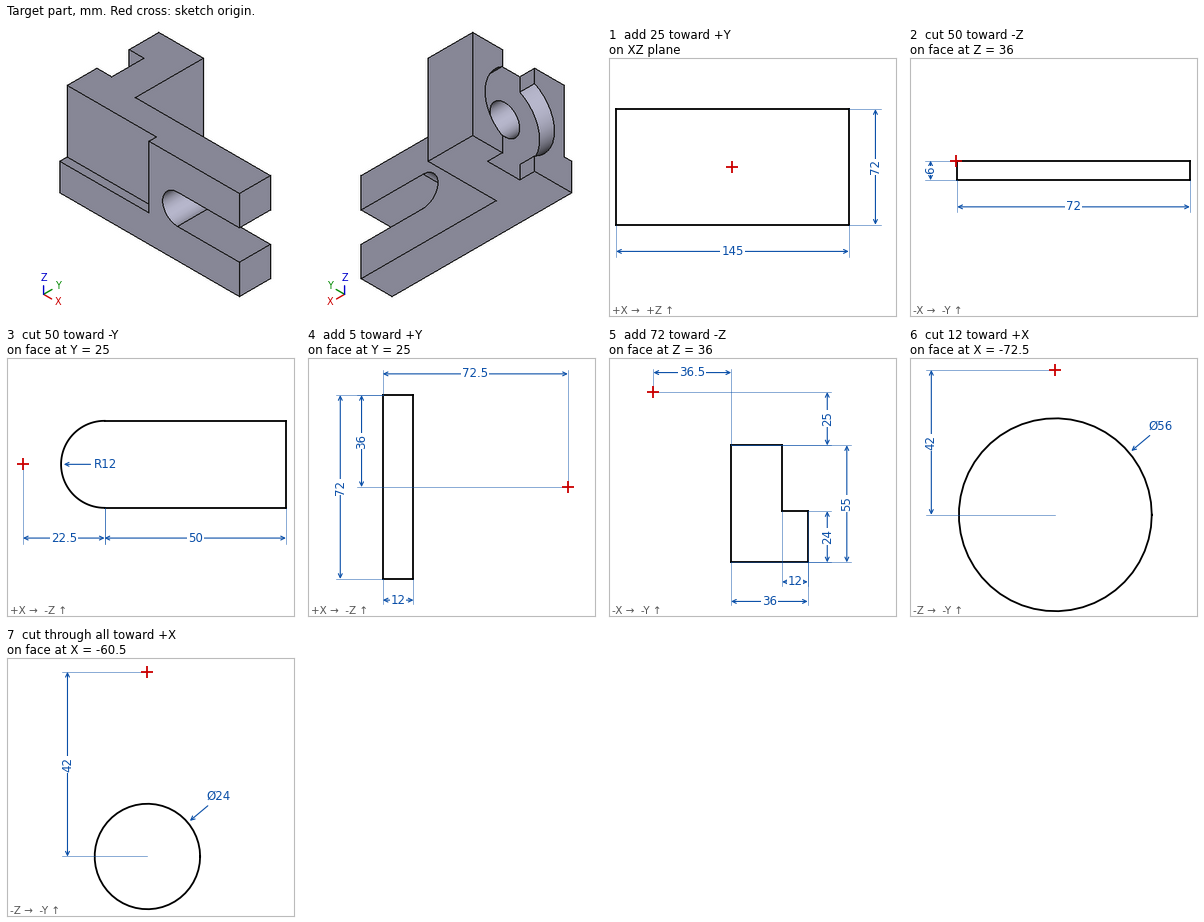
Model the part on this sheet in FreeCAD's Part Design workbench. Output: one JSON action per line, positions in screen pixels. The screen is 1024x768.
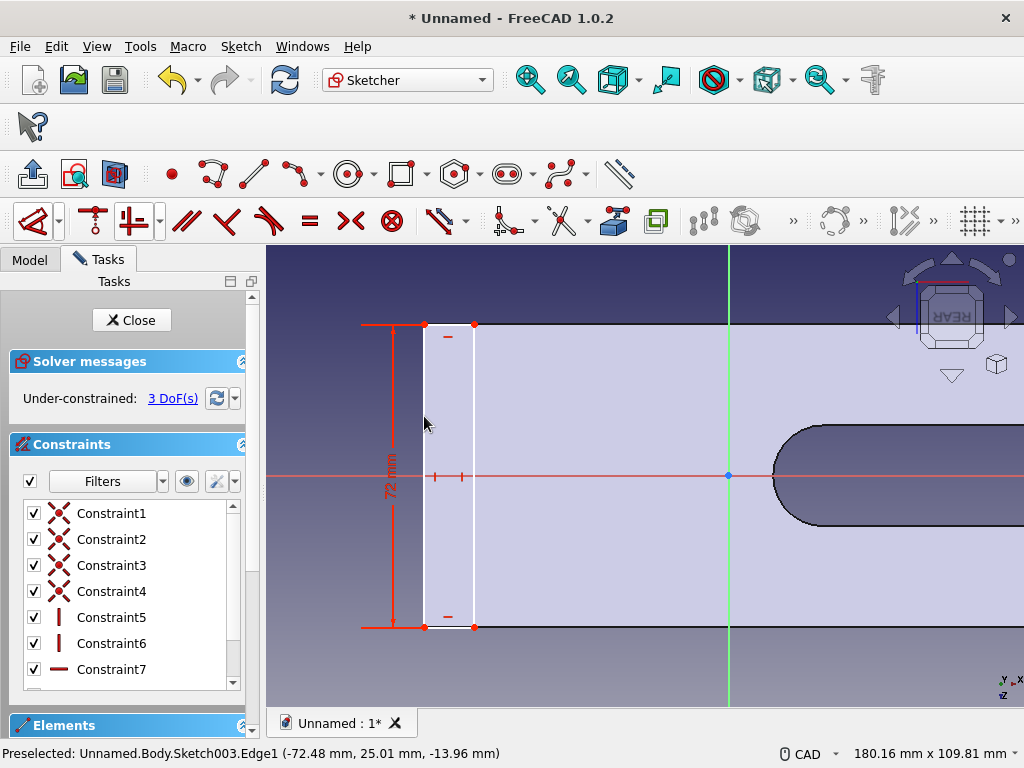
{"action": "left_click", "coordinate": [439, 628]}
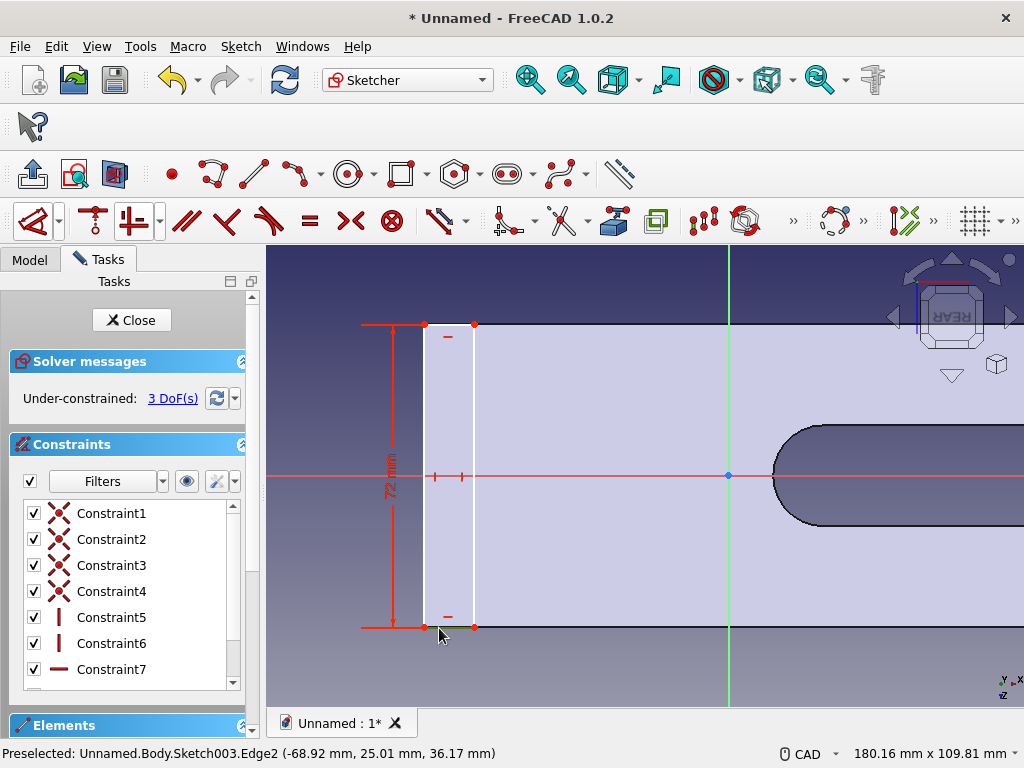
{"action": "key", "text": "l"}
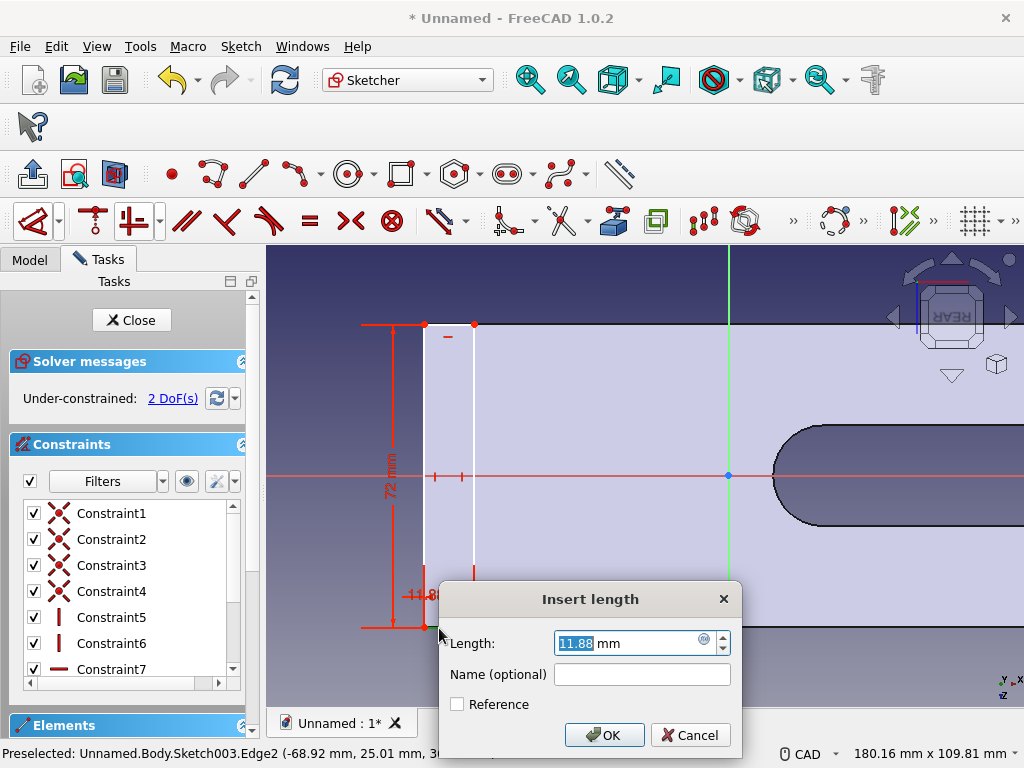
{"action": "type", "text": "12"}
{"action": "key", "text": "Return"}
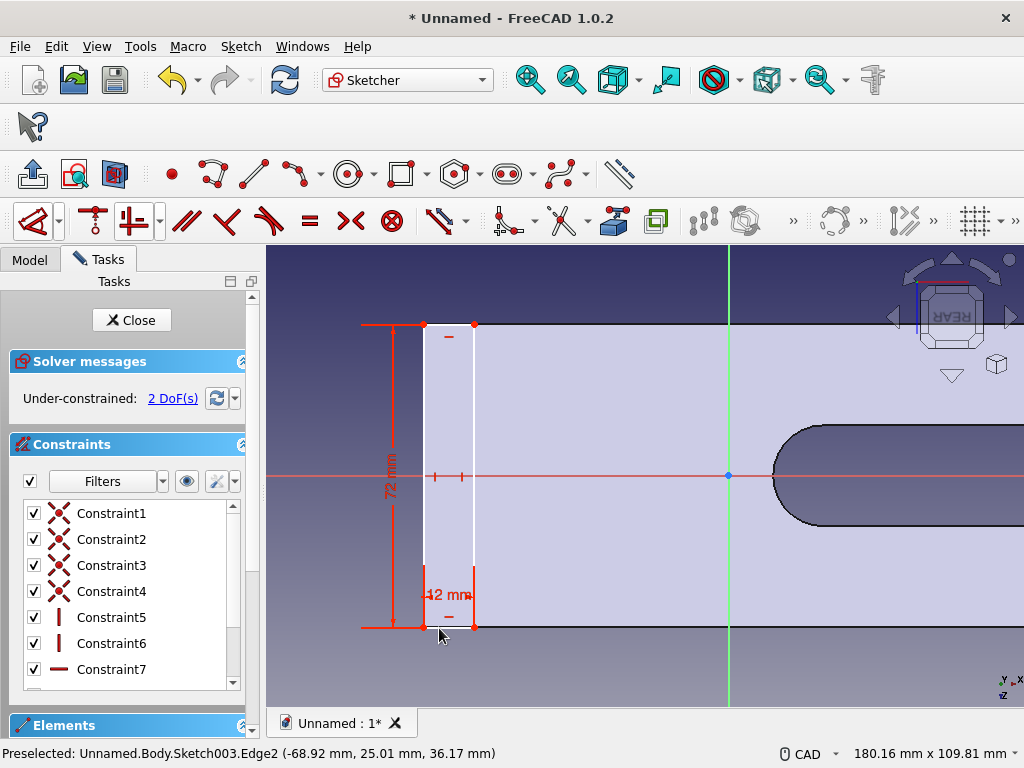
{"action": "left_click", "coordinate": [424, 325]}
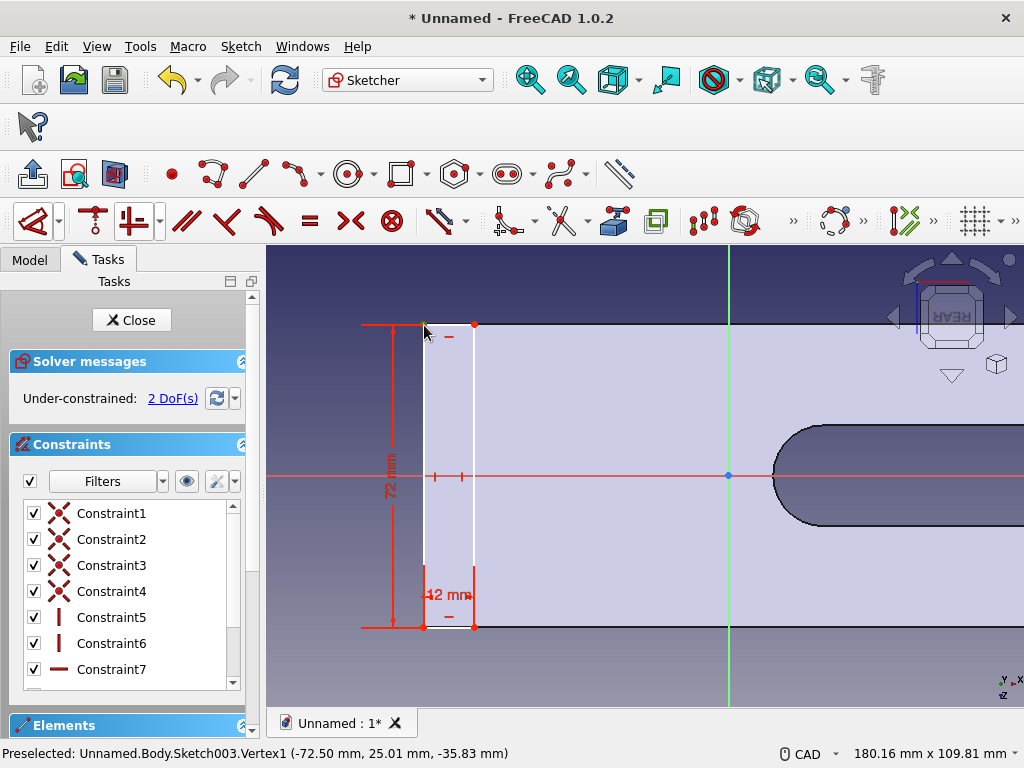
{"action": "left_click", "coordinate": [58, 222]}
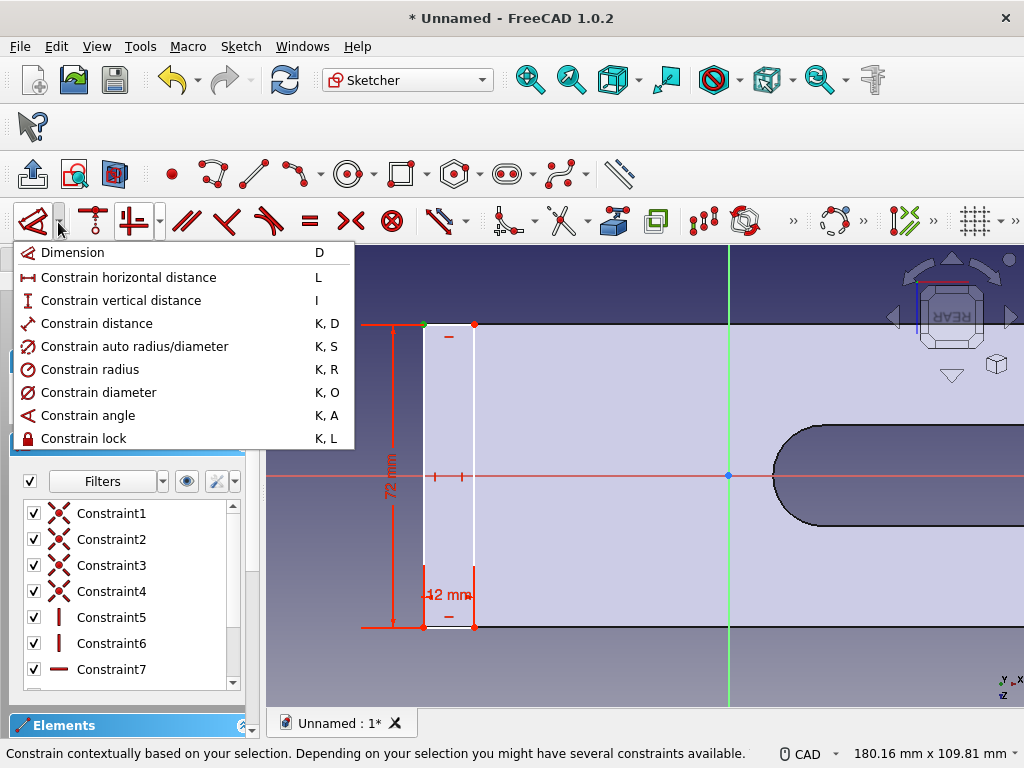
{"action": "left_click", "coordinate": [184, 300]}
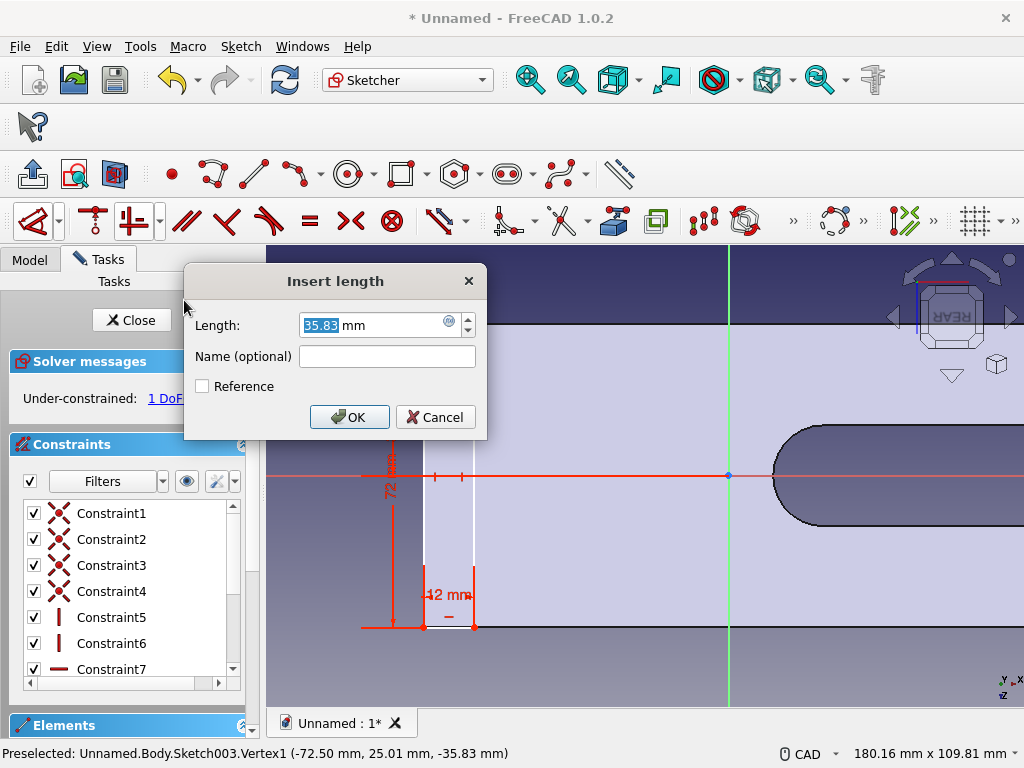
{"action": "type", "text": "36"}
{"action": "key", "text": "Return"}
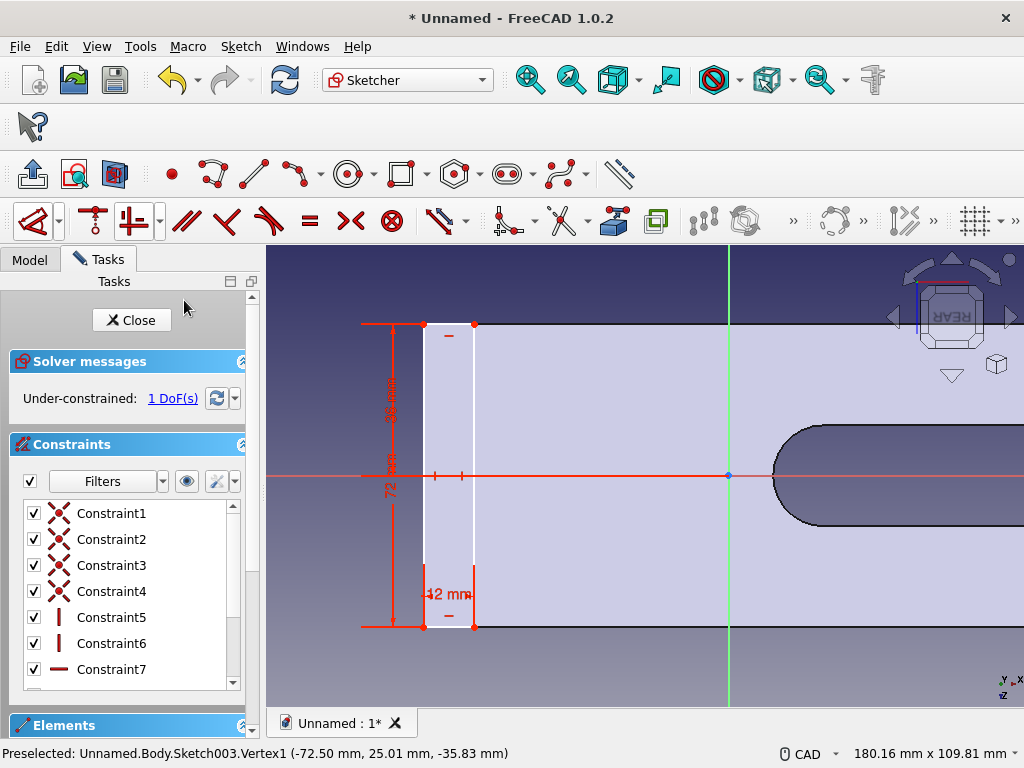
{"action": "left_click", "coordinate": [424, 324]}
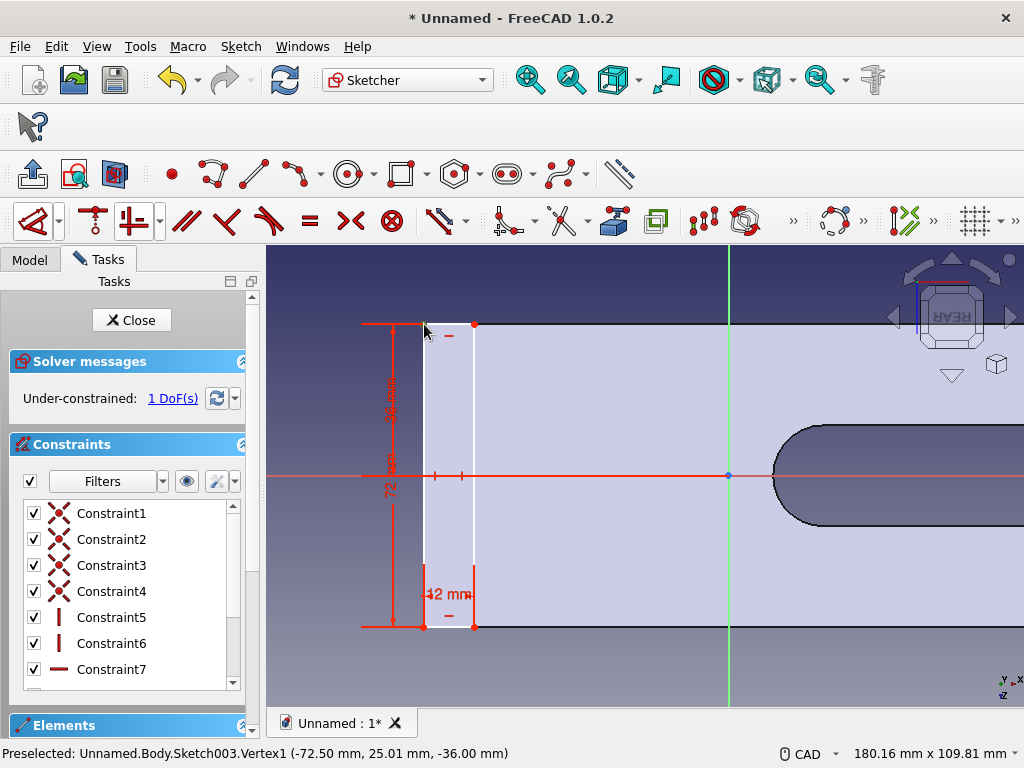
{"action": "key", "text": "l"}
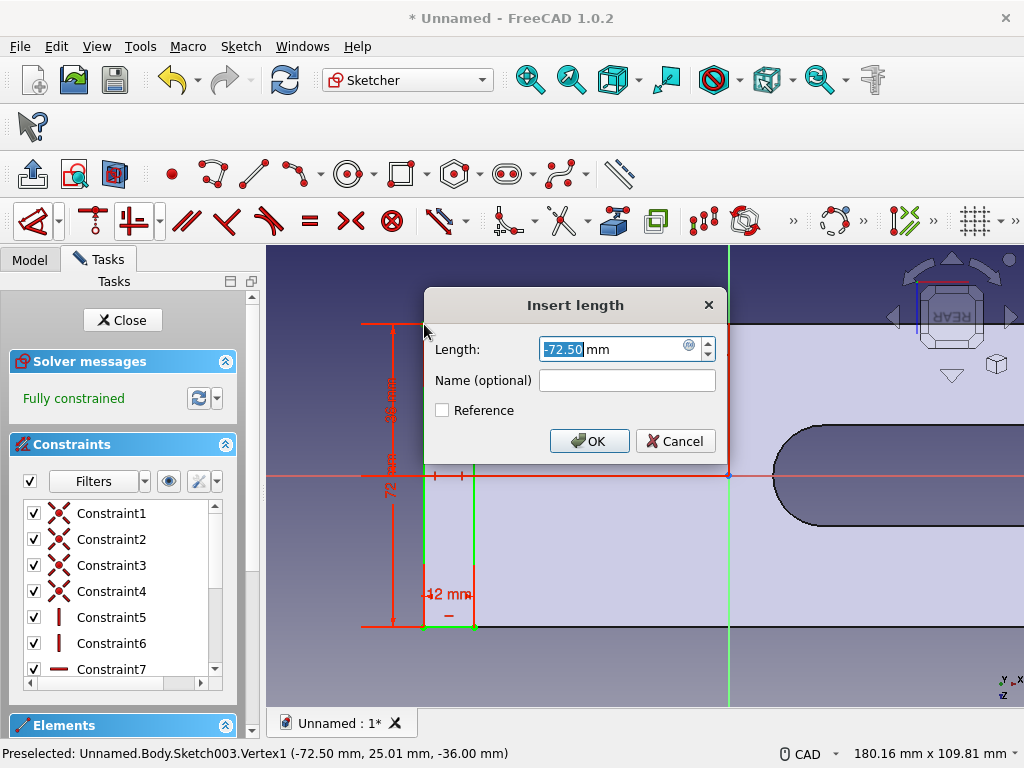
{"action": "type", "text": "-72.5"}
{"action": "key", "text": "Return"}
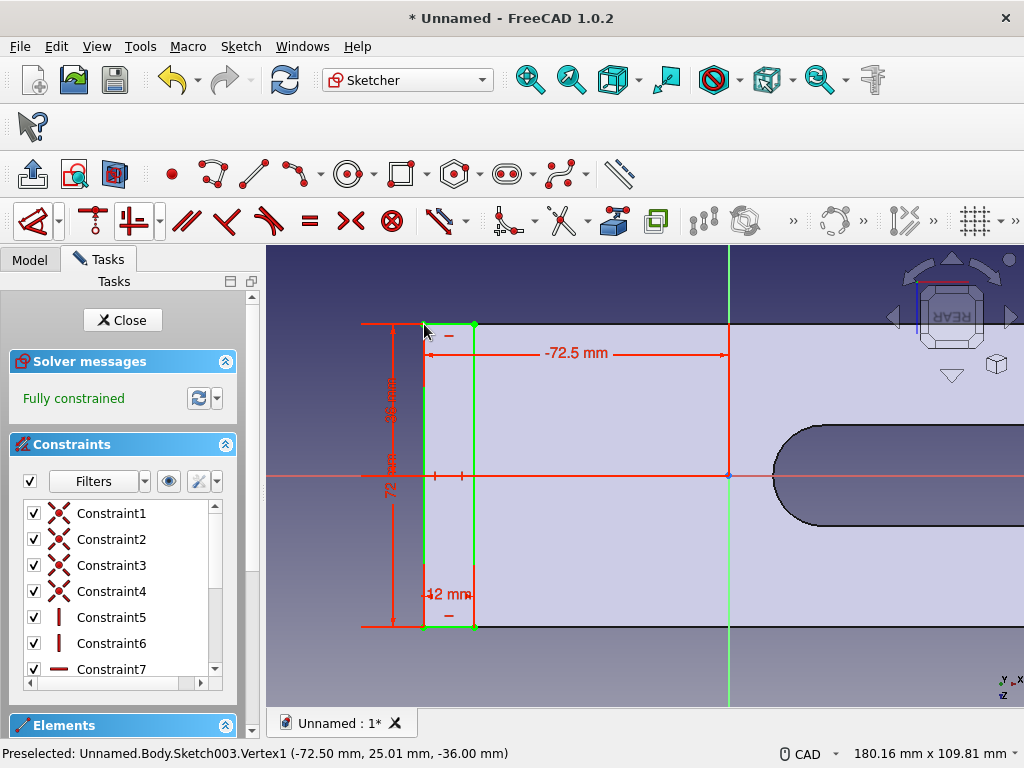
{"action": "left_click", "coordinate": [123, 320]}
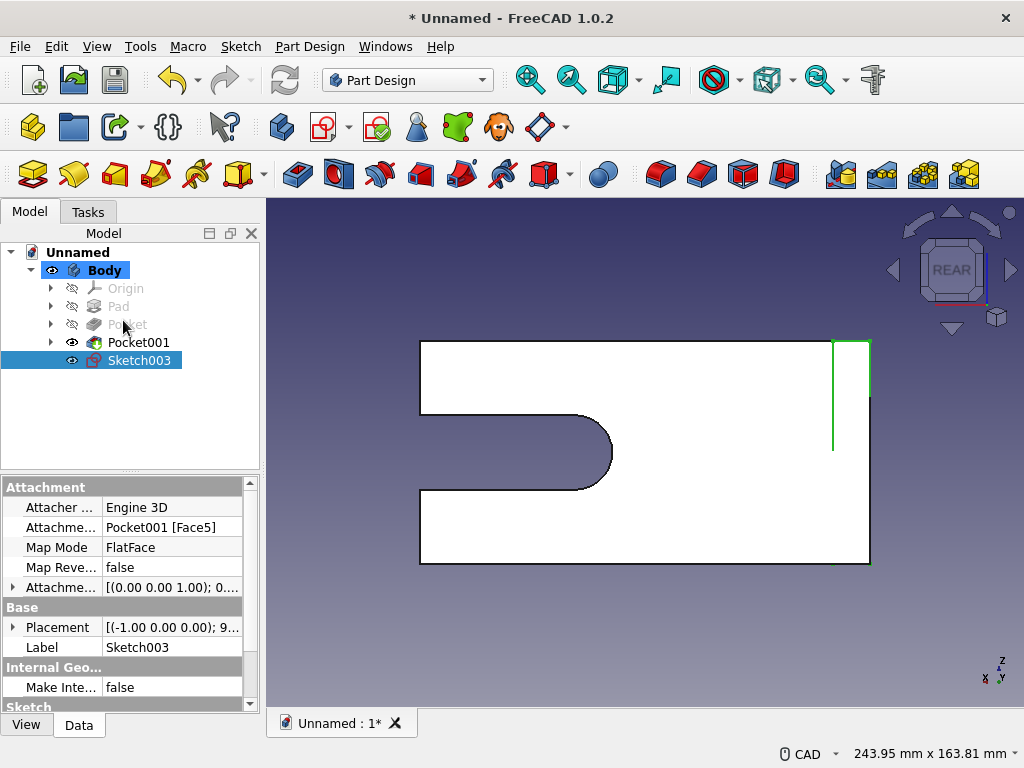
{"action": "left_click", "coordinate": [33, 174]}